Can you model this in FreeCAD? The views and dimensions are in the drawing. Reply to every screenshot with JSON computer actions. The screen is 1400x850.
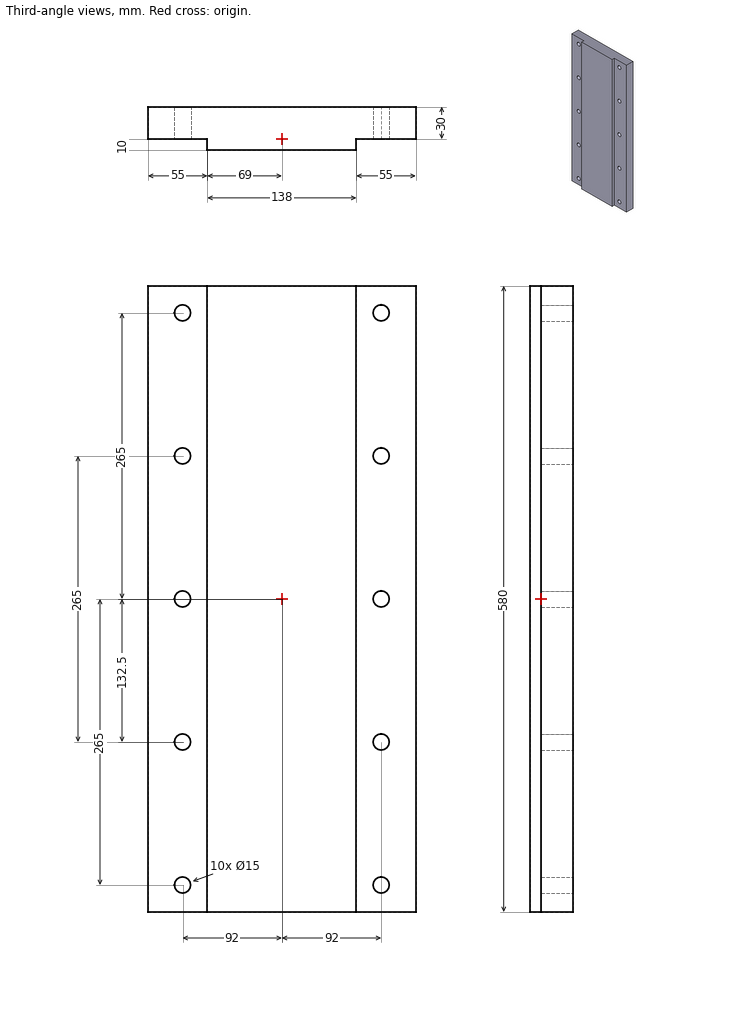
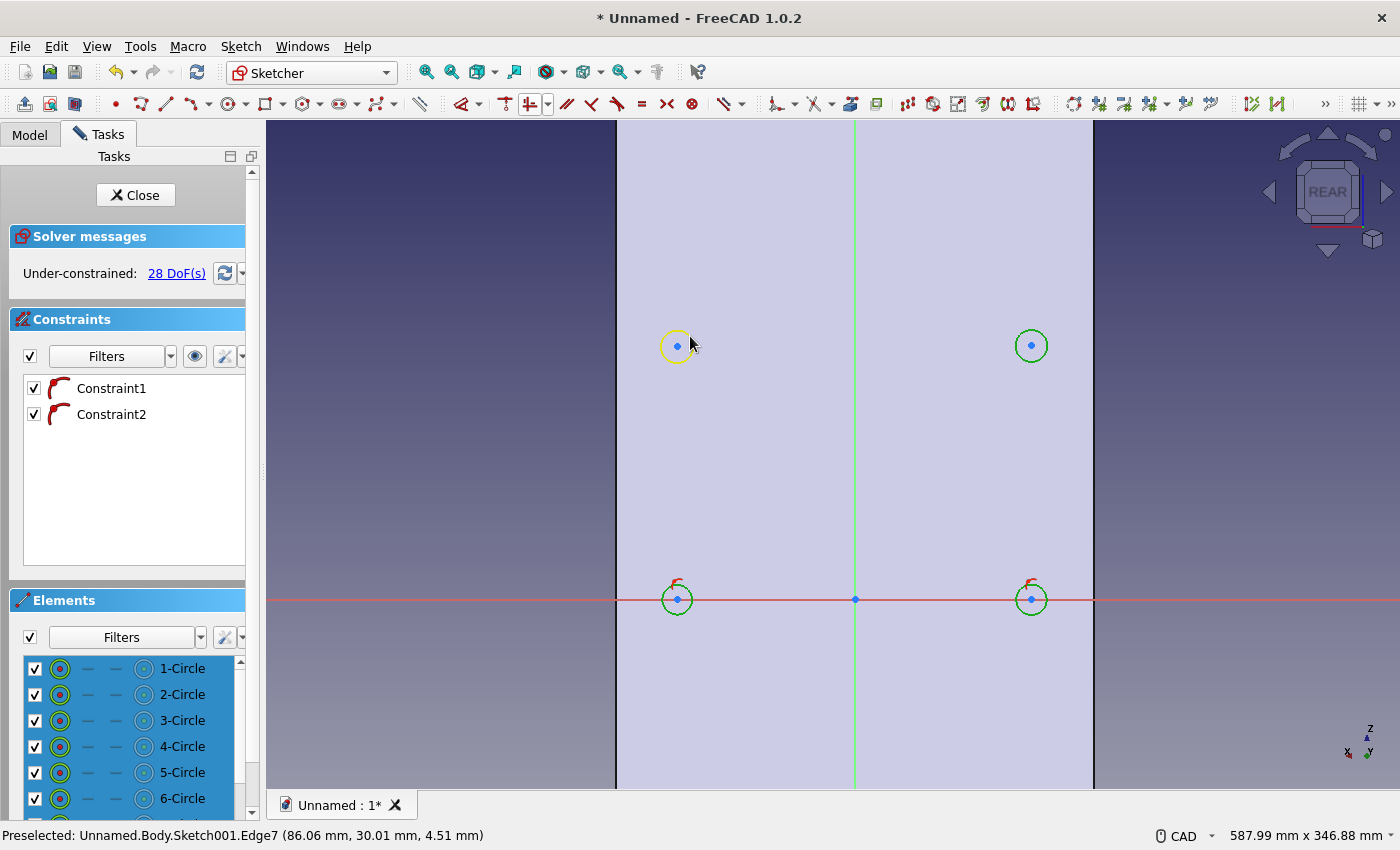
{"action": "left_click", "coordinate": [689, 335]}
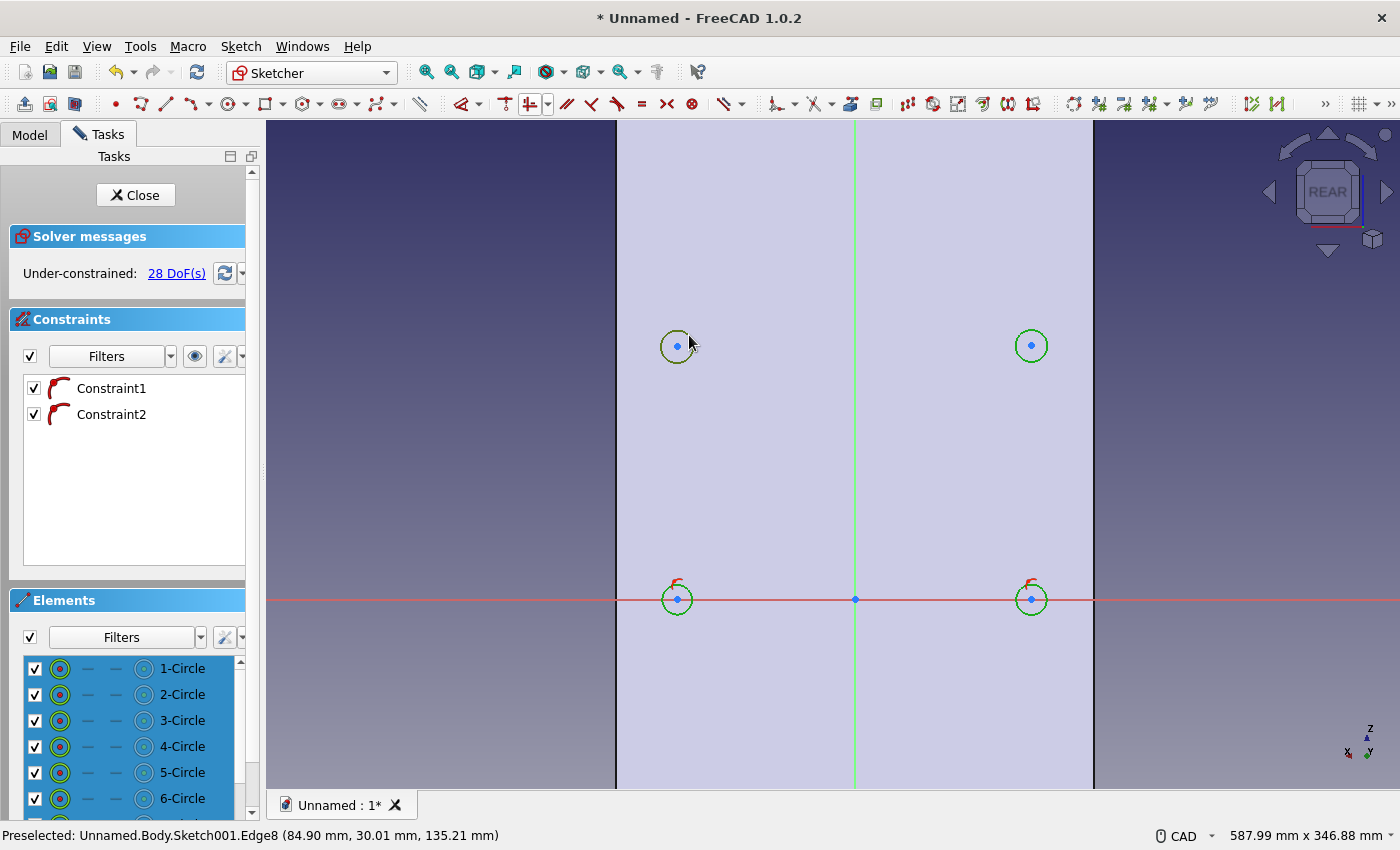
{"action": "scroll", "coordinate": [691, 336], "scroll_direction": "down", "scroll_amount": 4}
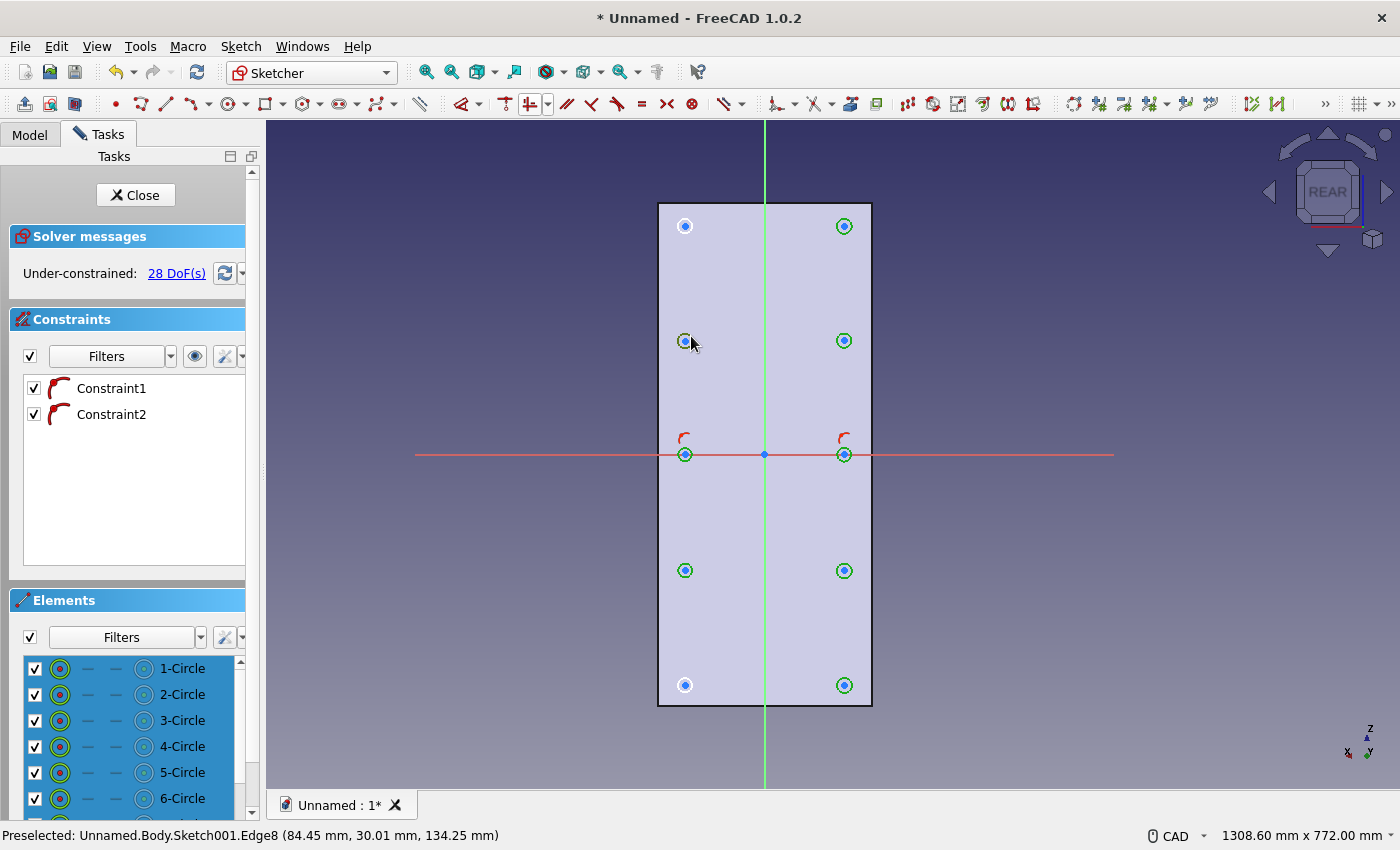
{"action": "scroll", "coordinate": [690, 221], "scroll_direction": "up", "scroll_amount": 4}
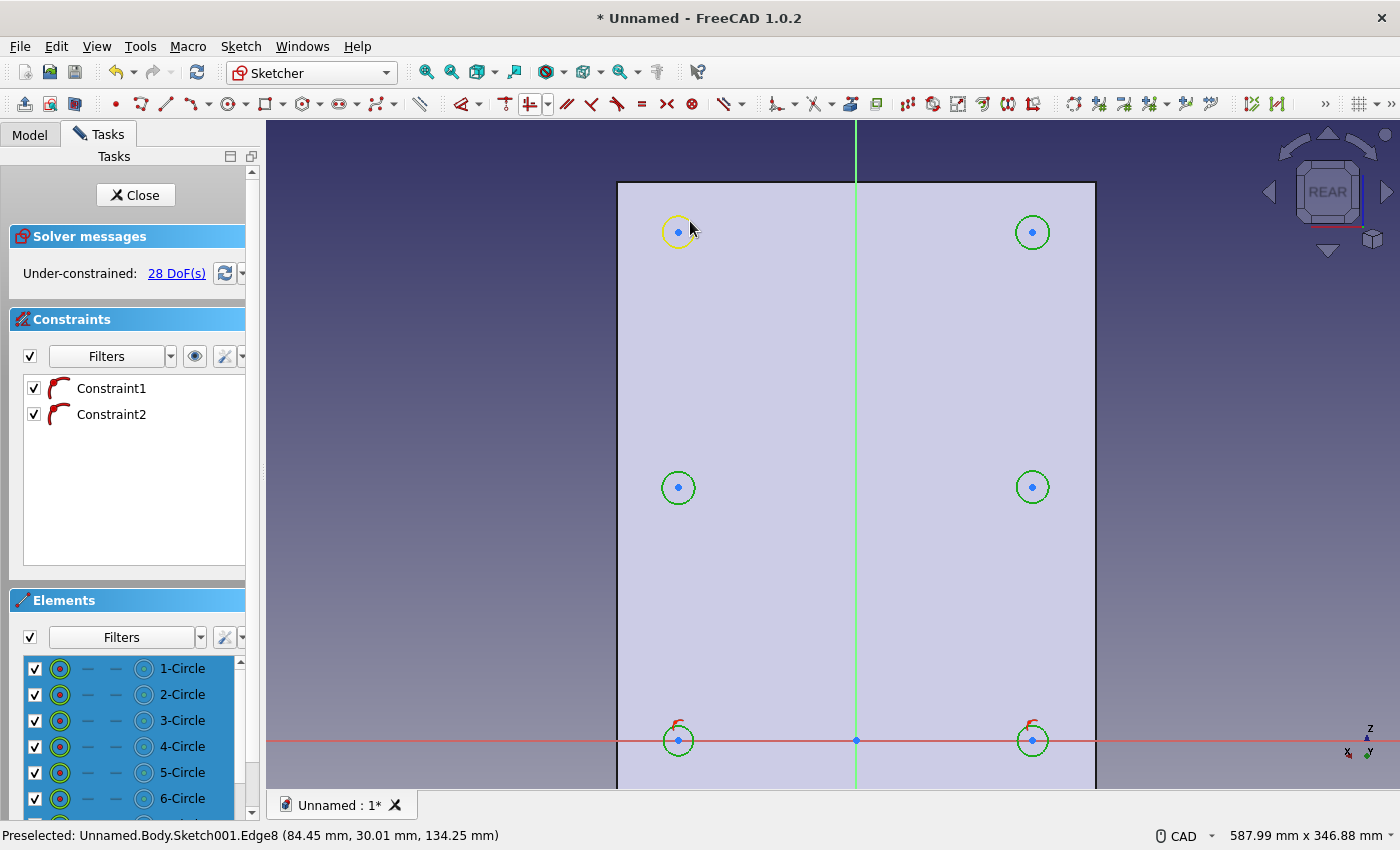
{"action": "left_click", "coordinate": [690, 221]}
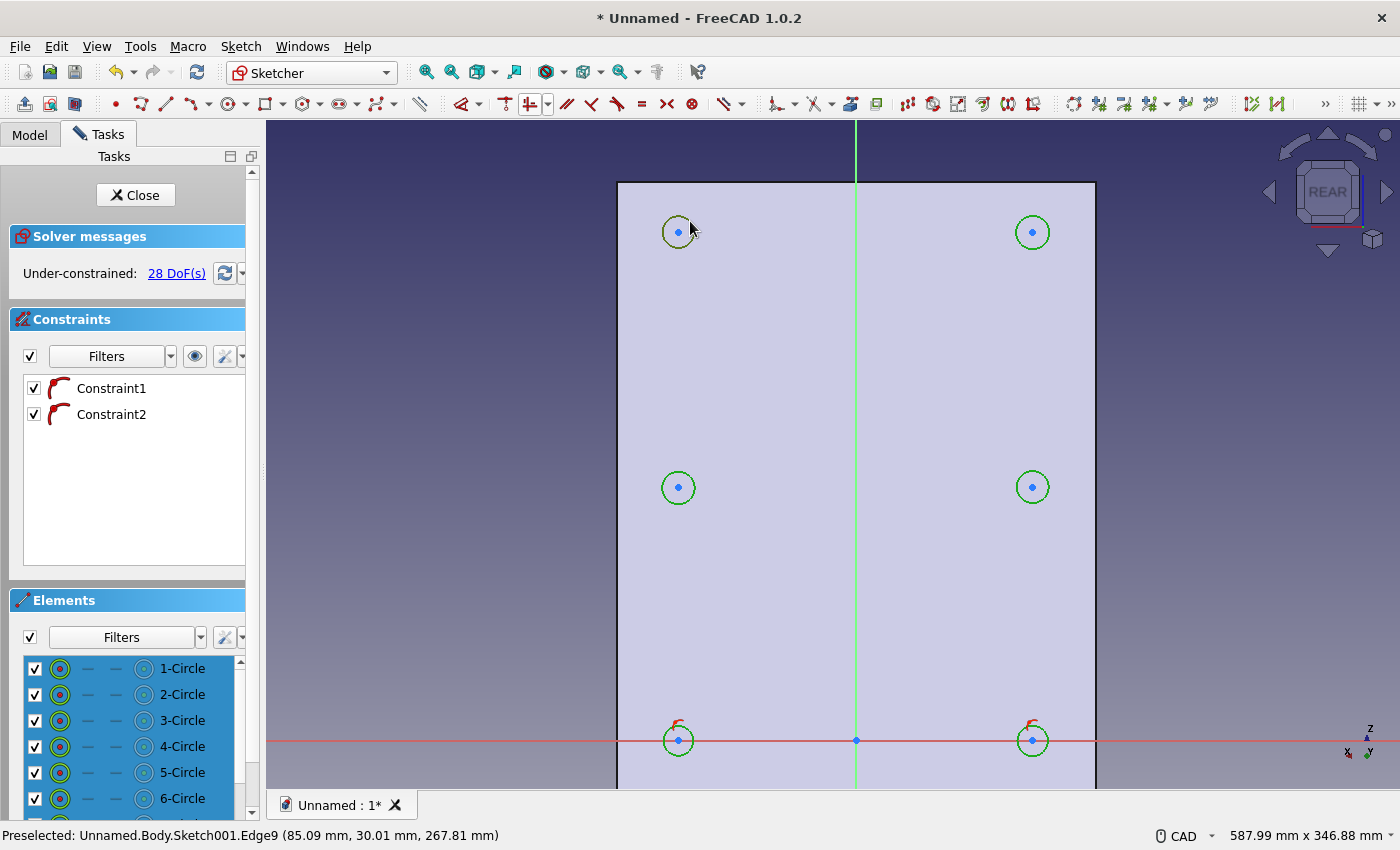
{"action": "scroll", "coordinate": [690, 221], "scroll_direction": "down", "scroll_amount": 4}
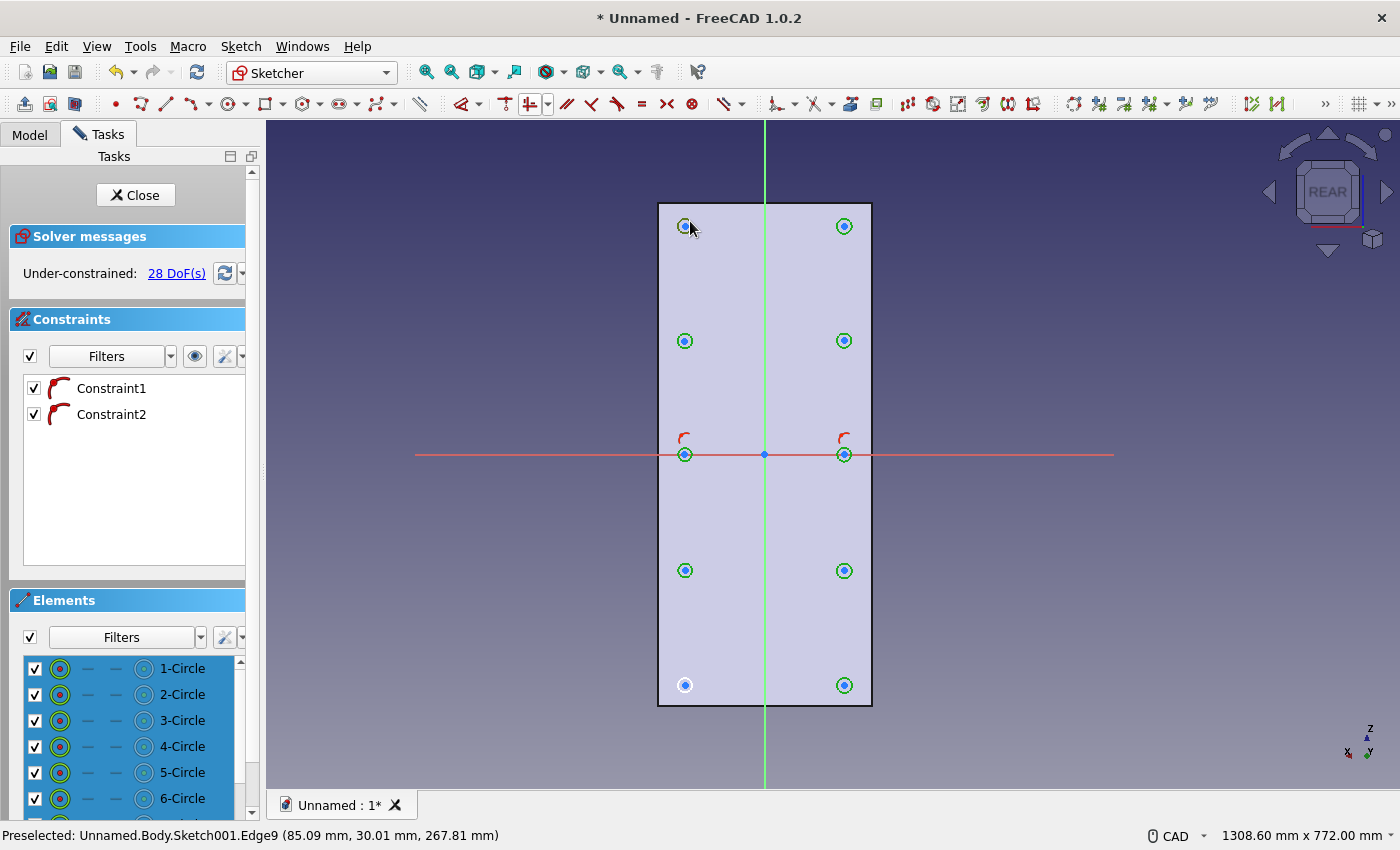
{"action": "scroll", "coordinate": [690, 680], "scroll_direction": "up", "scroll_amount": 4}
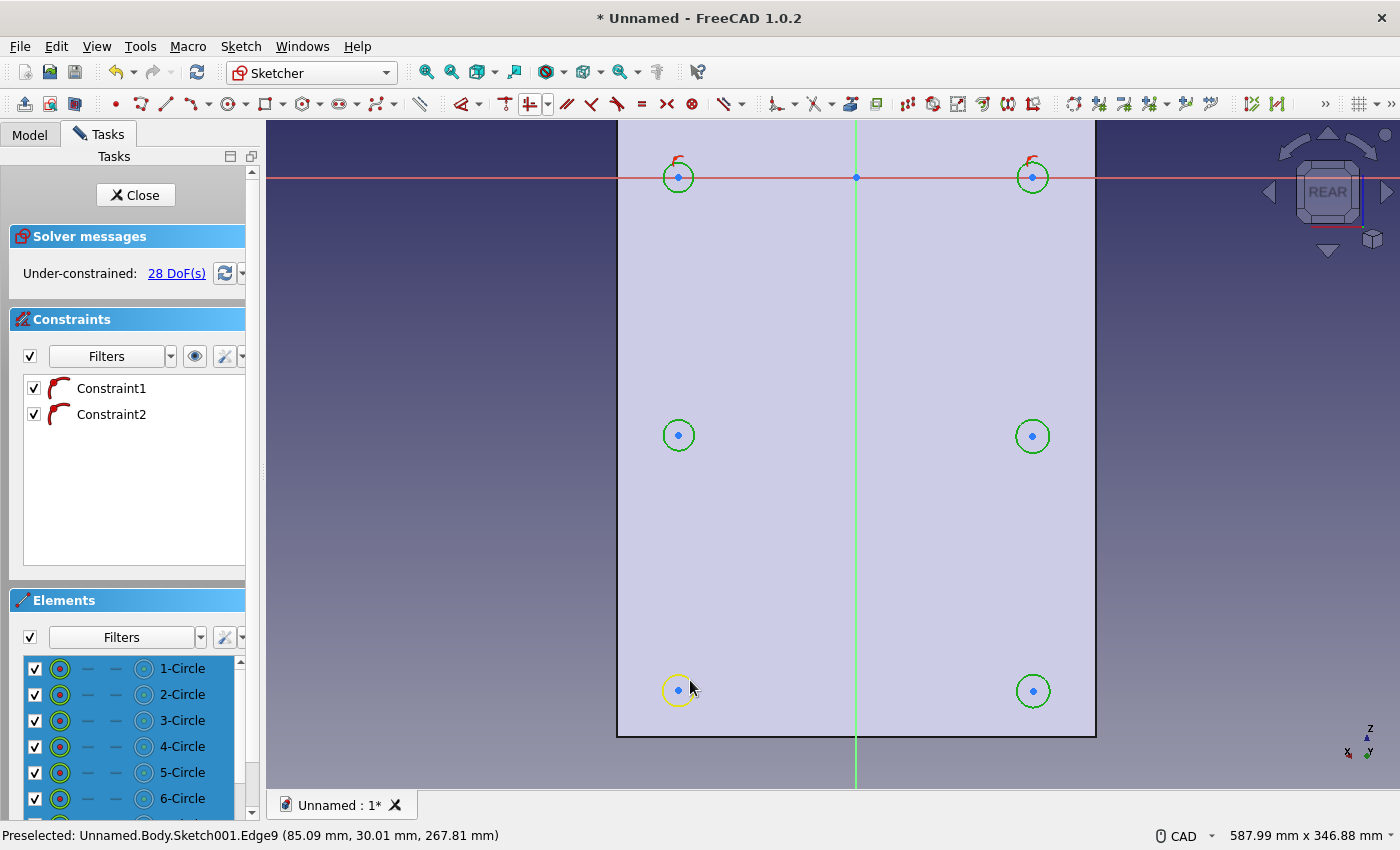
{"action": "left_click", "coordinate": [689, 680]}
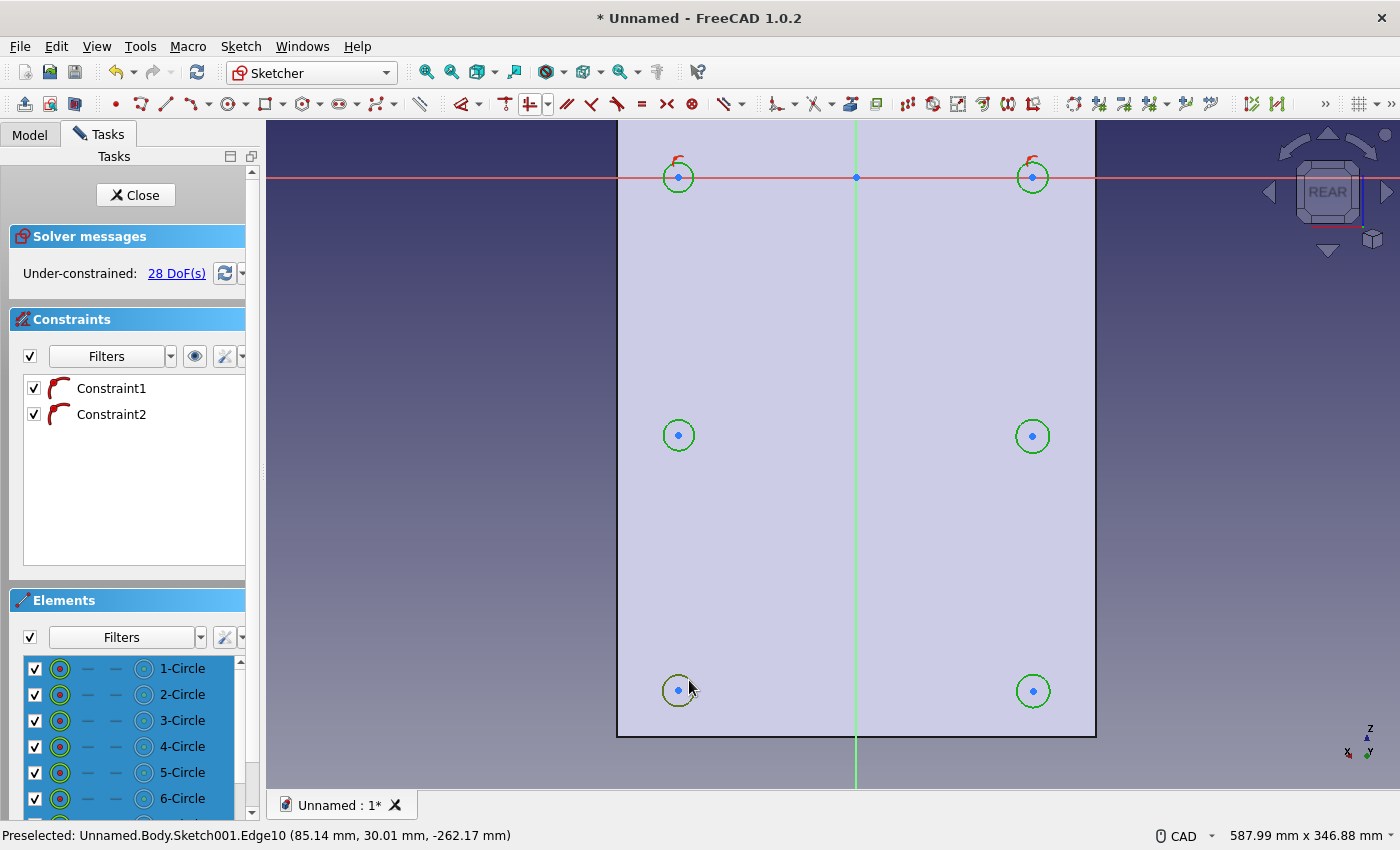
{"action": "key", "text": "e"}